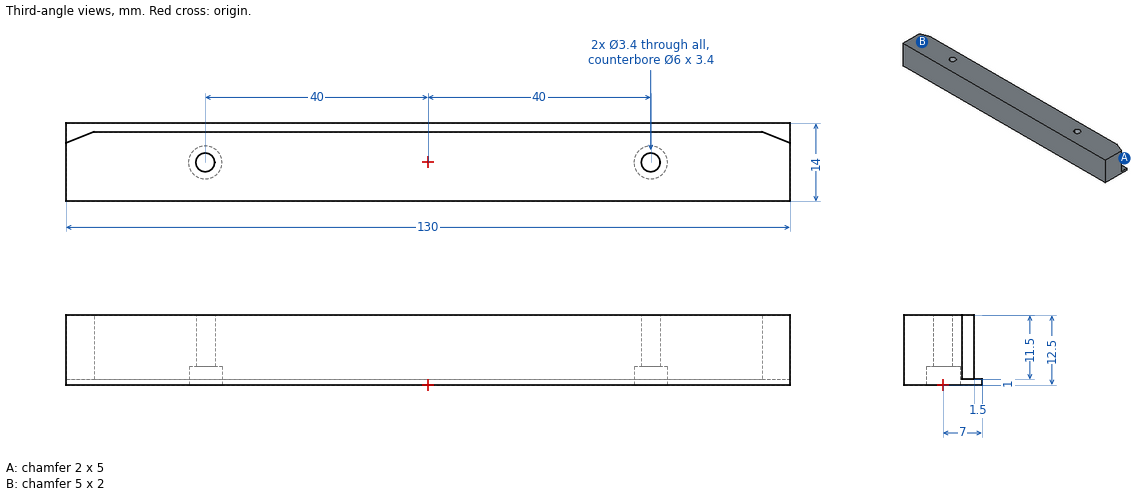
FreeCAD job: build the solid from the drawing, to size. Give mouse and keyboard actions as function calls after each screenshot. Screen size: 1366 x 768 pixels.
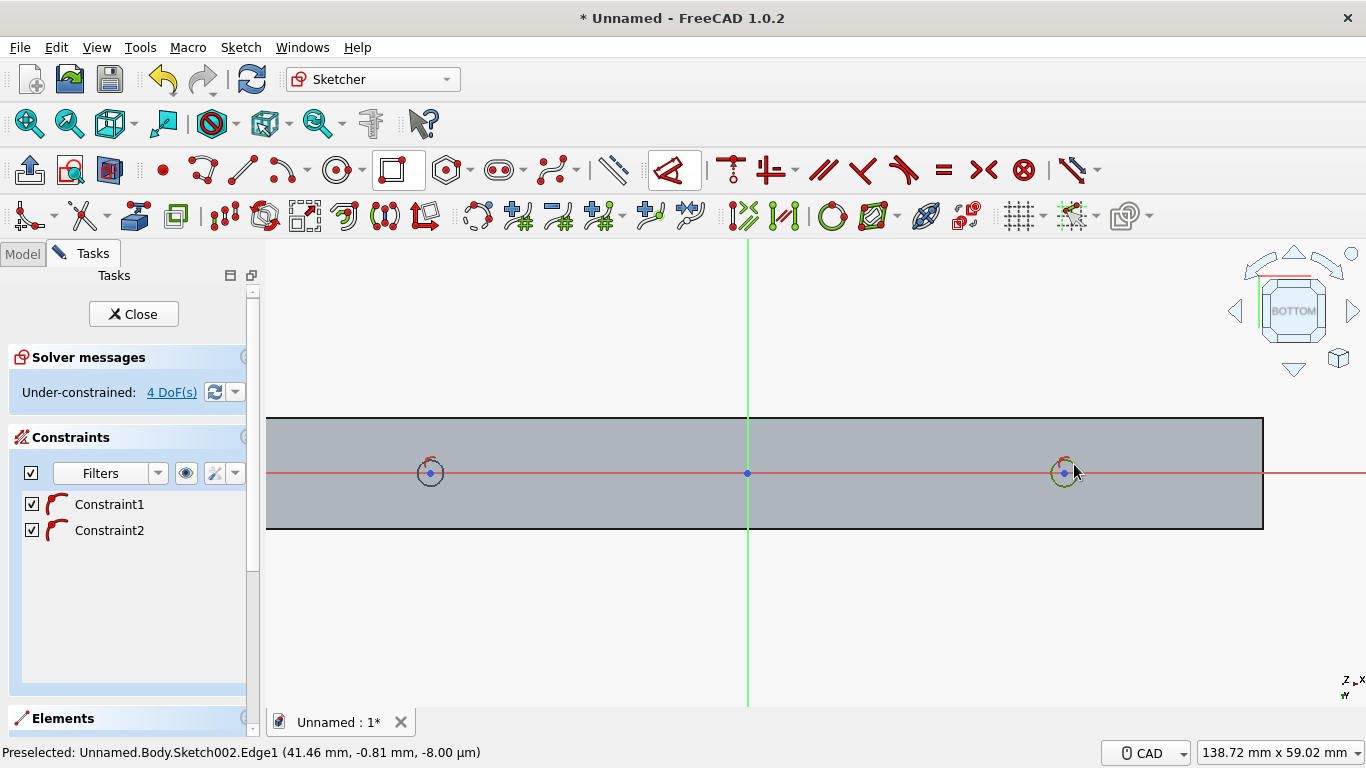
scroll(440, 464, up, 3)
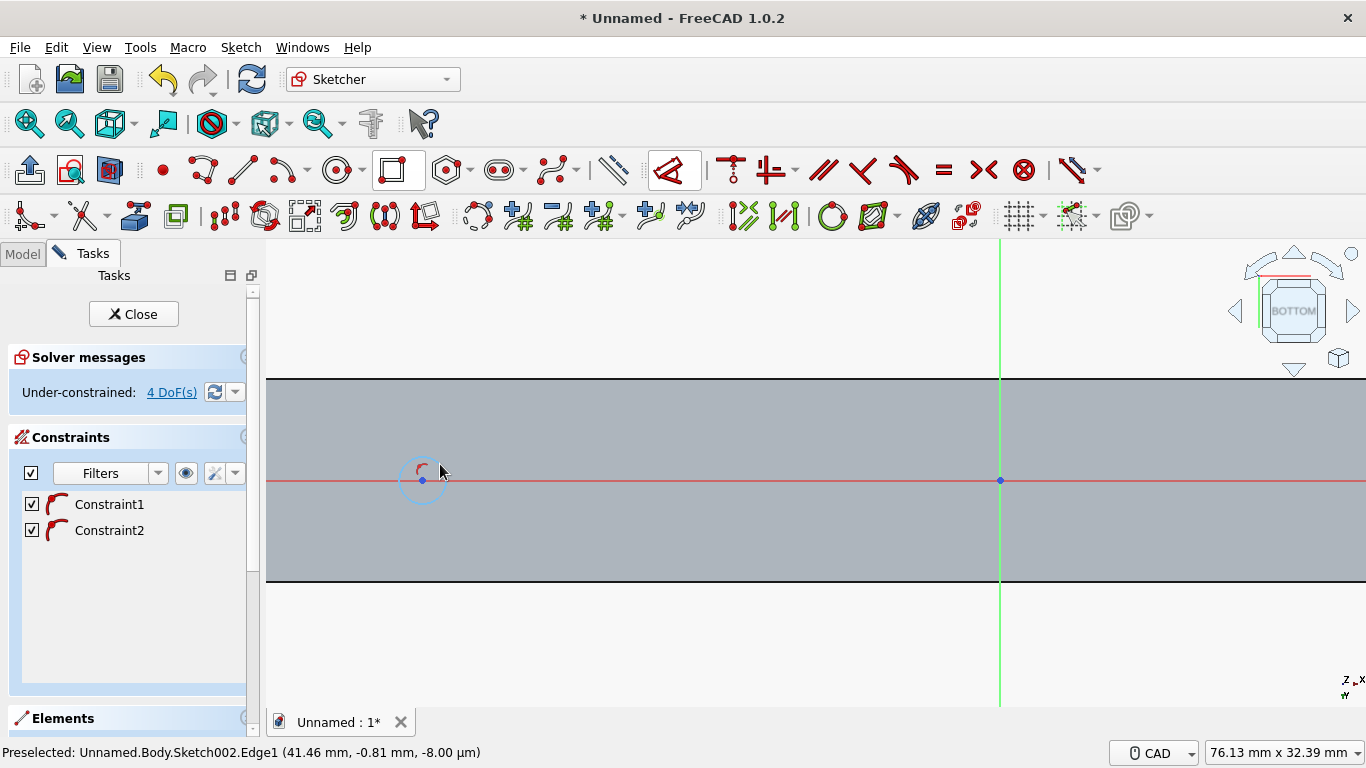
click(439, 464)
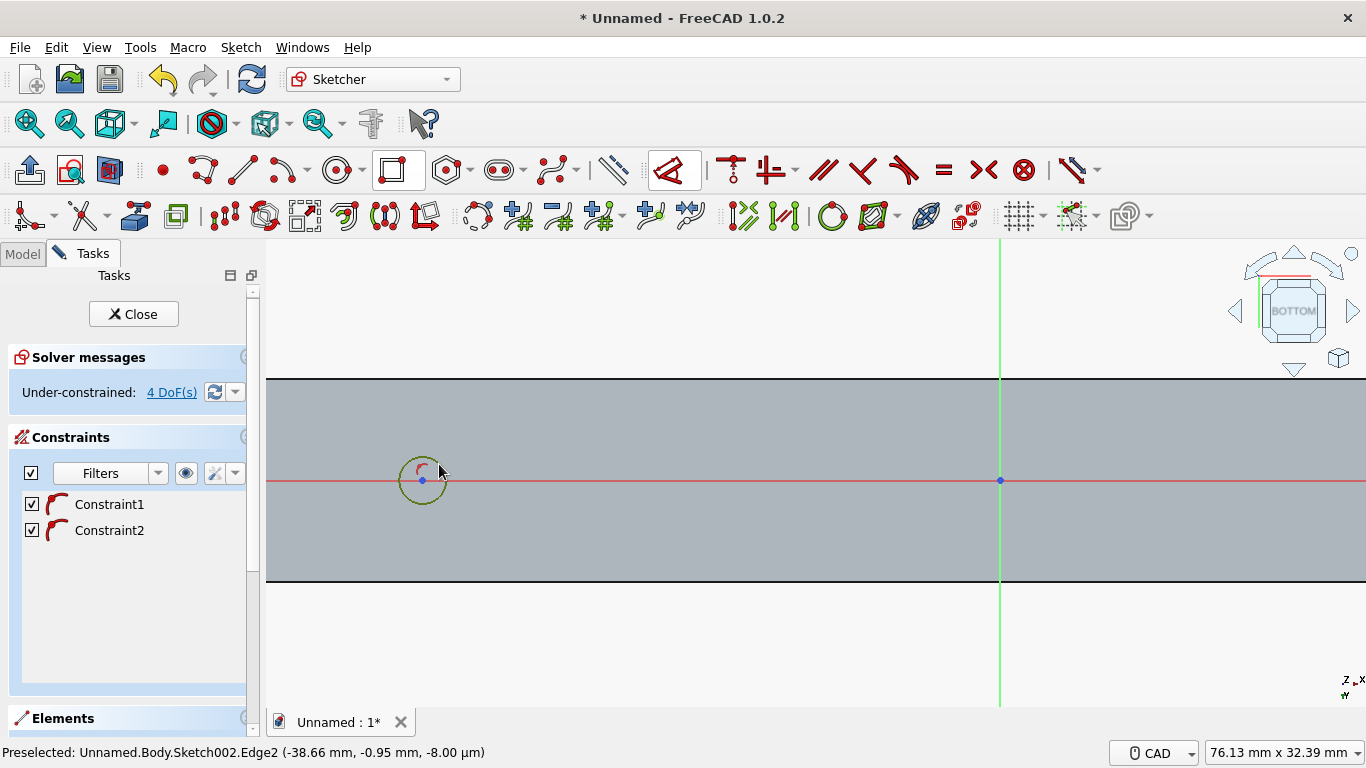
click(944, 170)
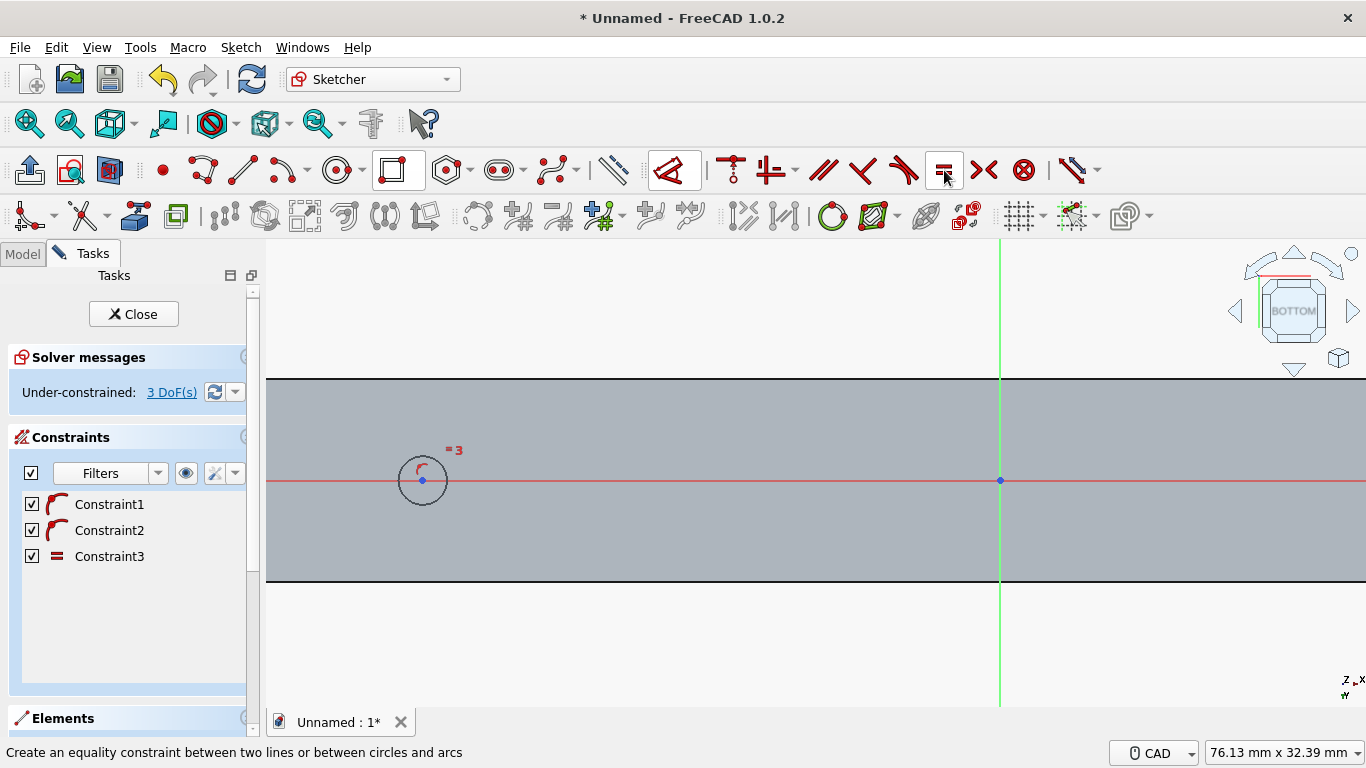
scroll(440, 464, down, 3)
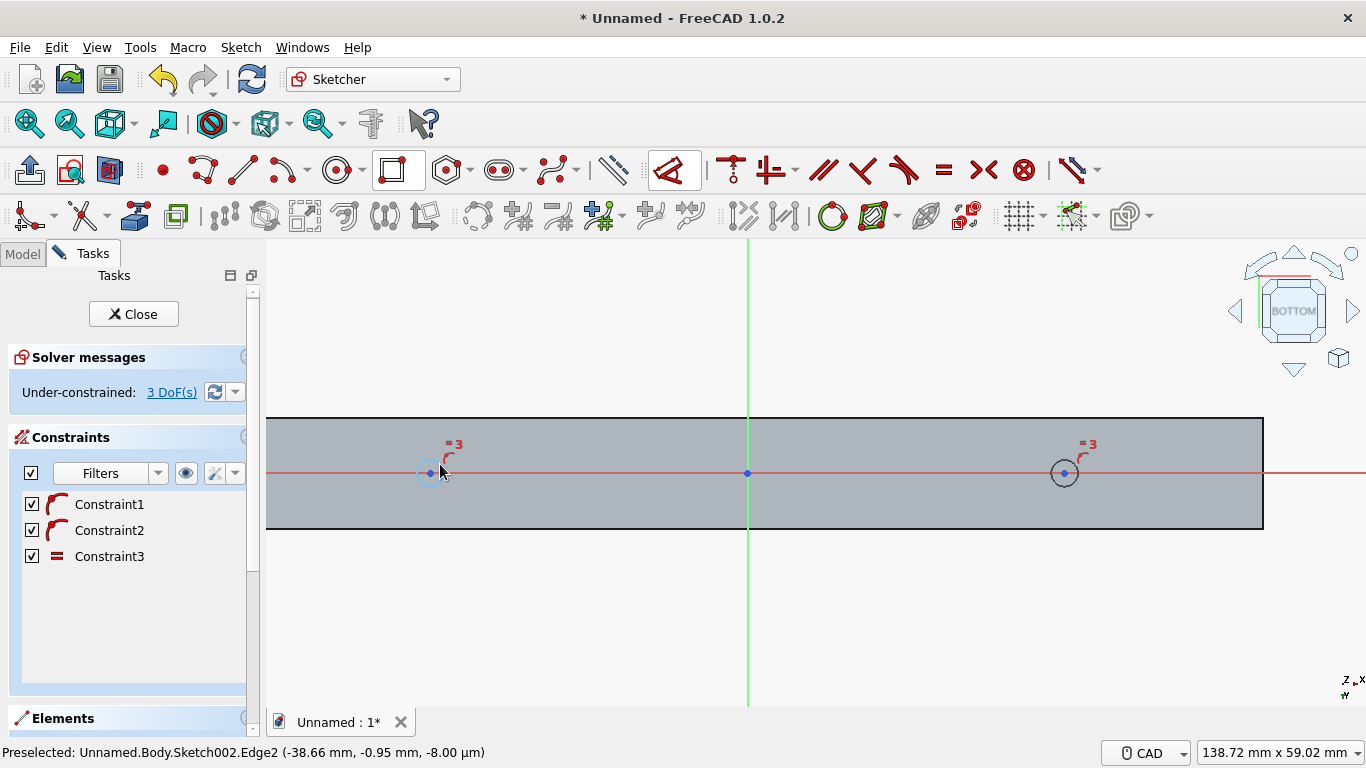
scroll(1074, 464, up, 2)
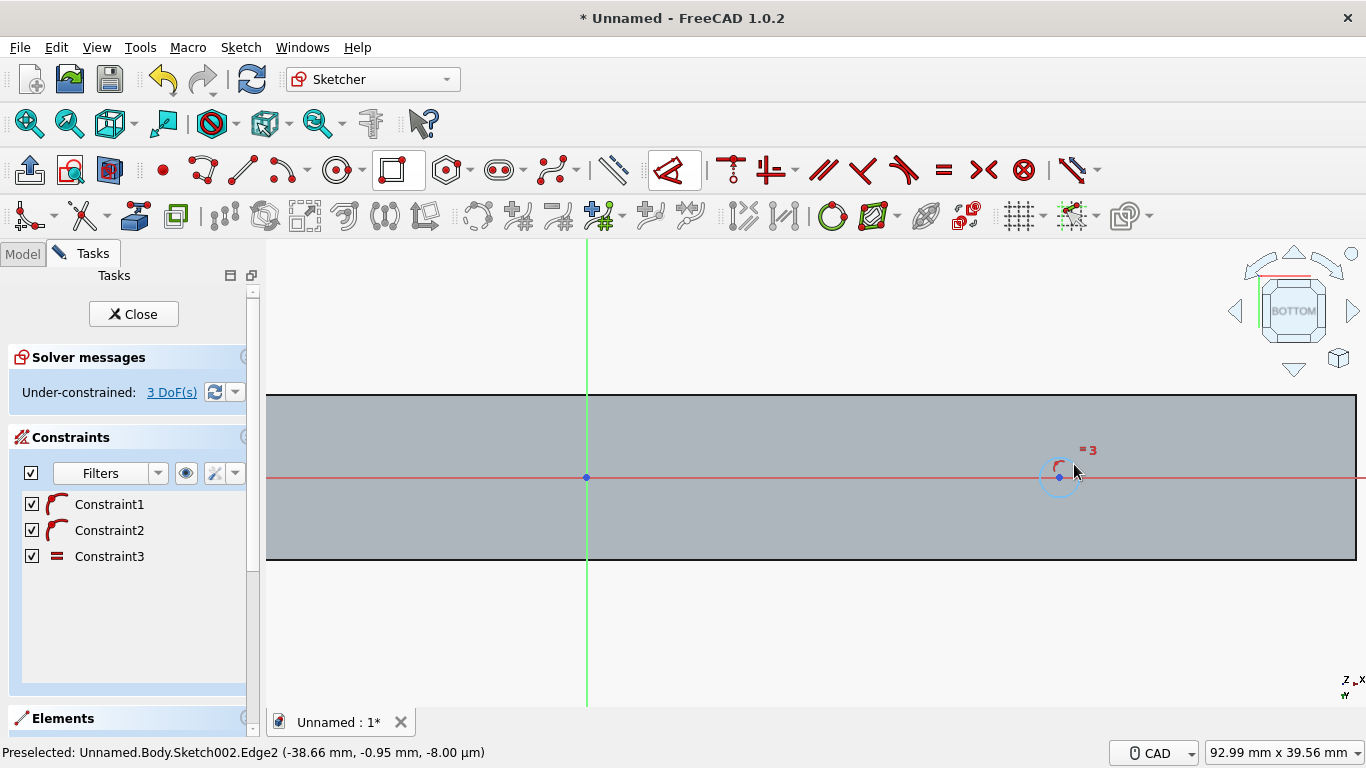
click(1074, 464)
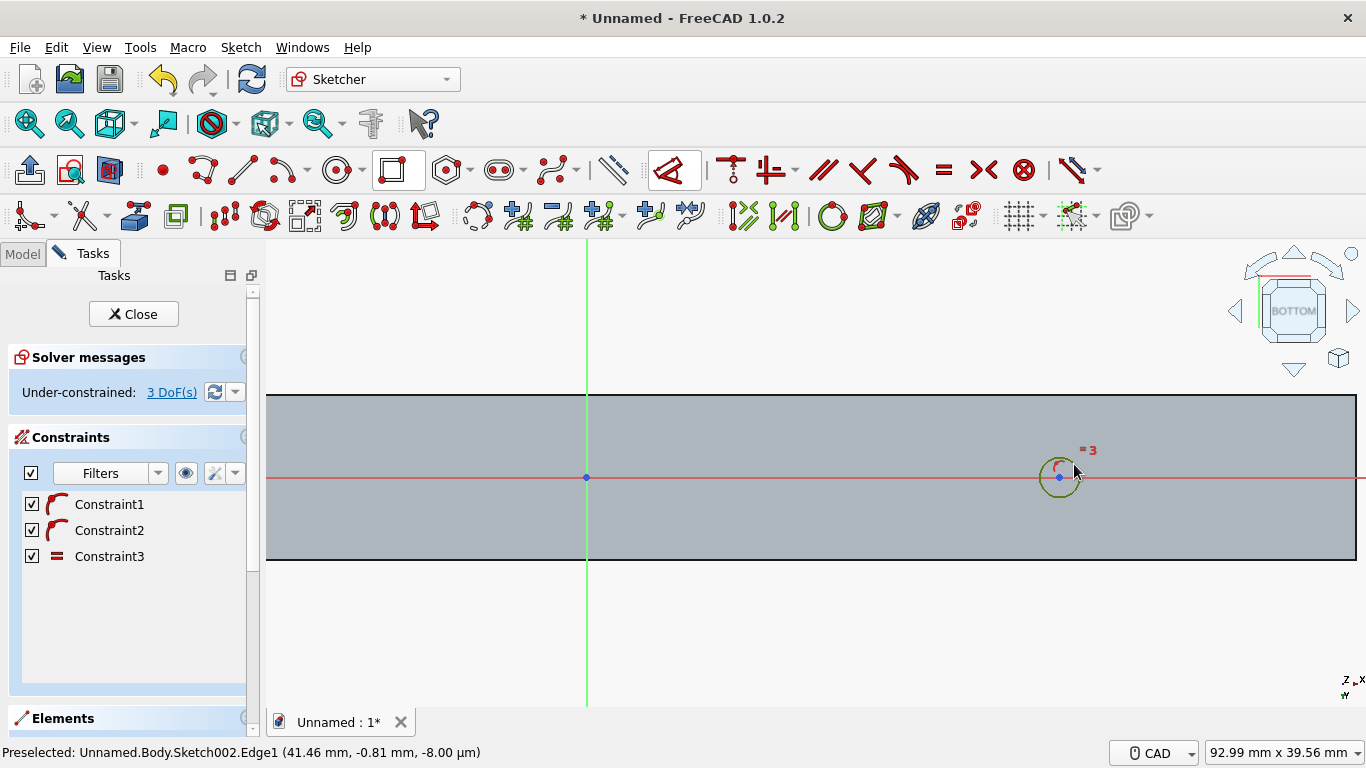
key(k)
key(o)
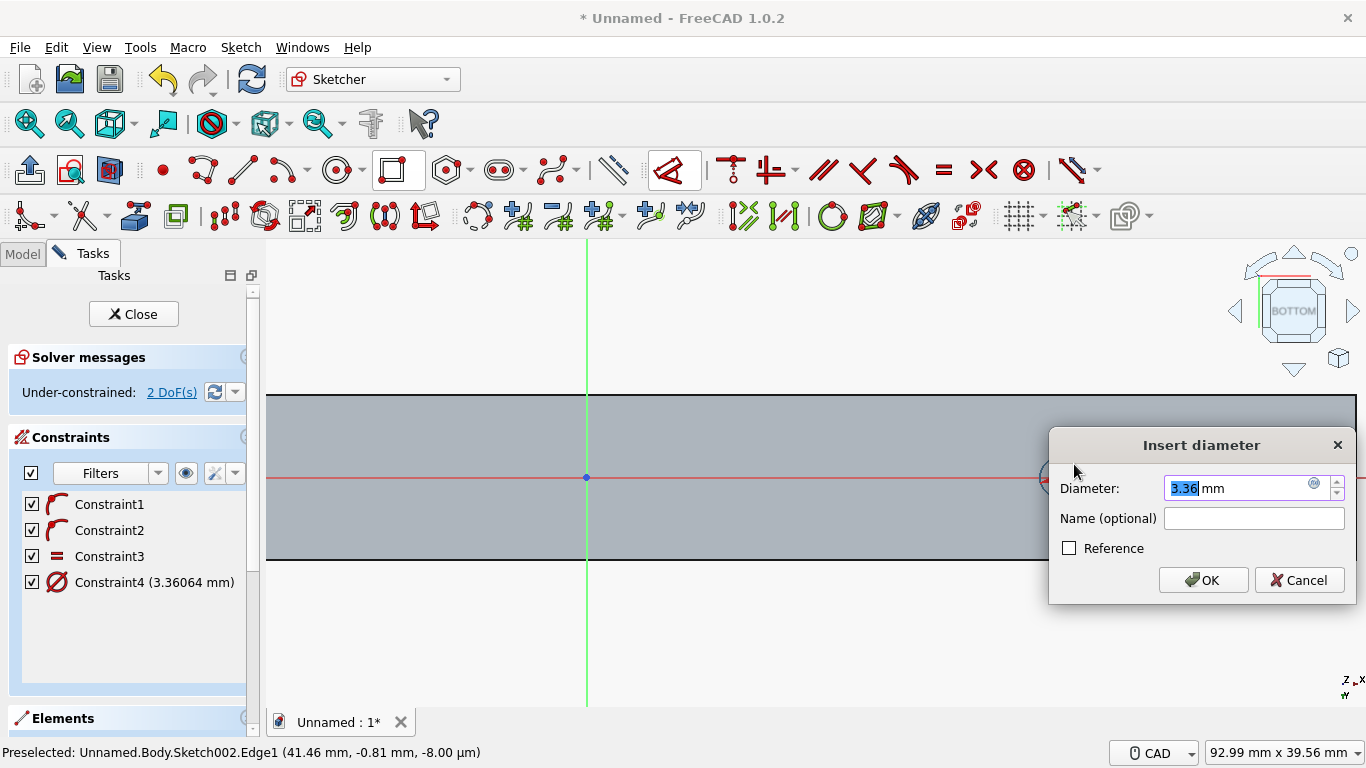
text(3.4)
key(Return)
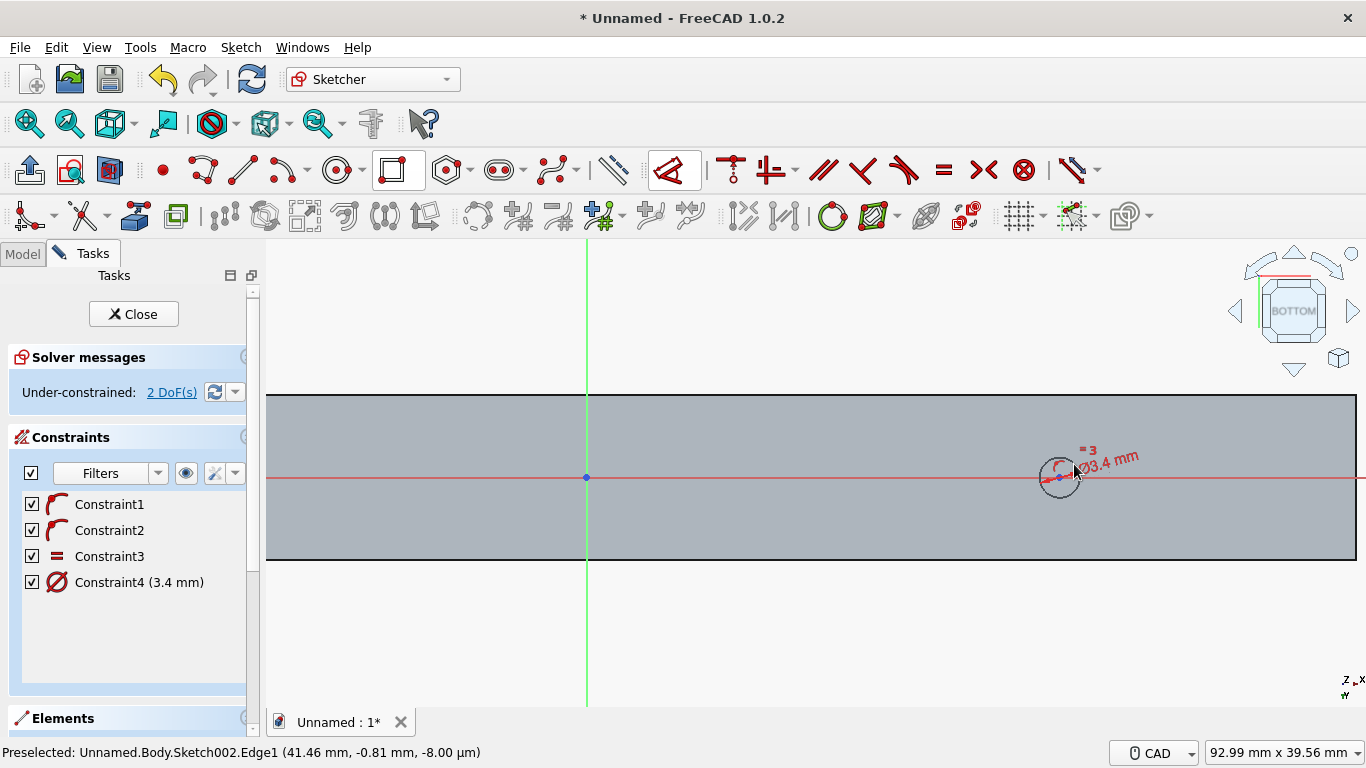
click(1060, 478)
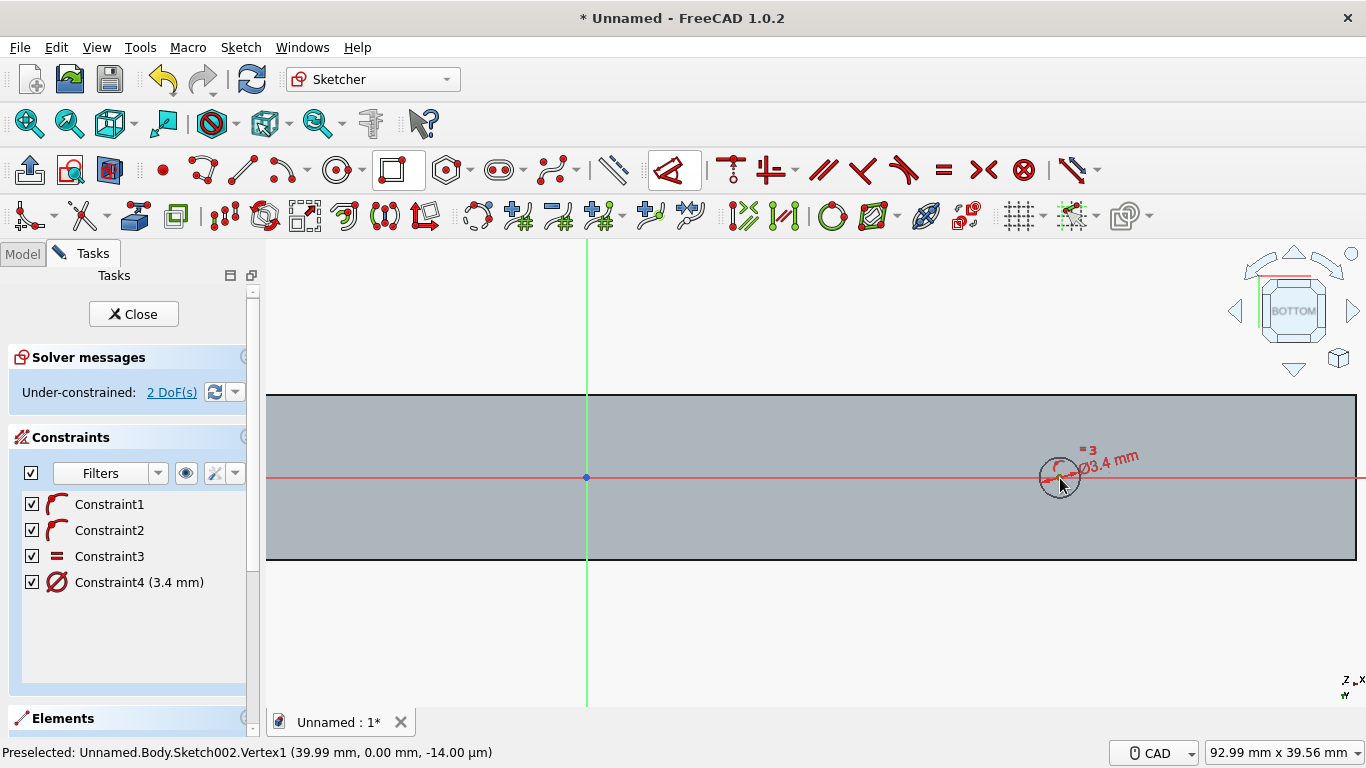
key(l)